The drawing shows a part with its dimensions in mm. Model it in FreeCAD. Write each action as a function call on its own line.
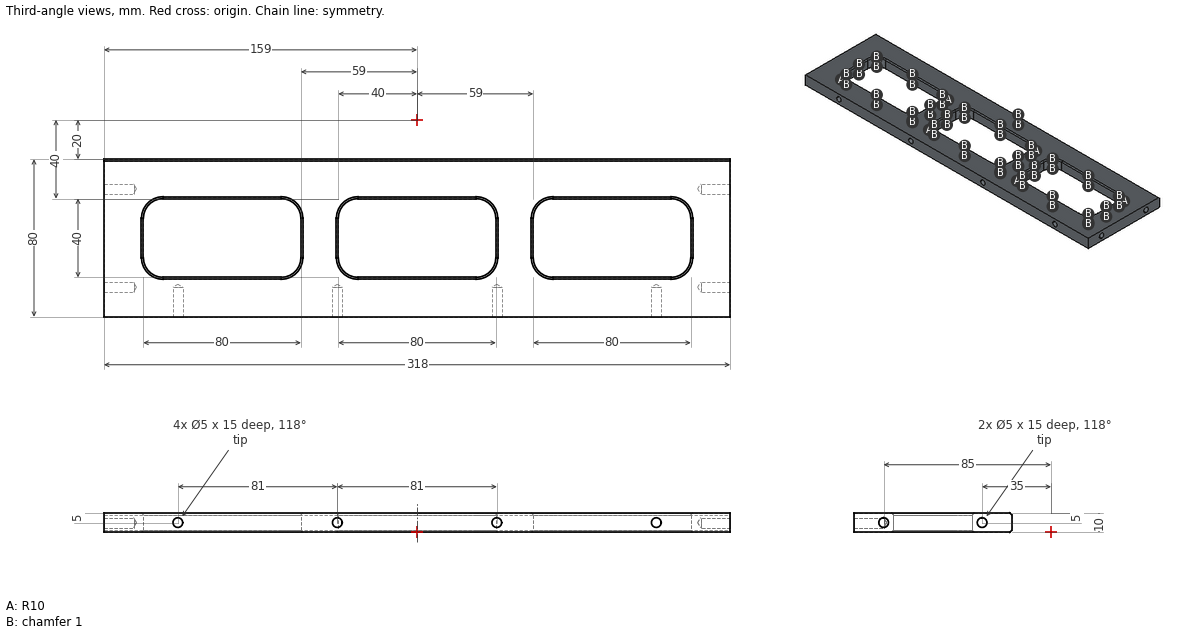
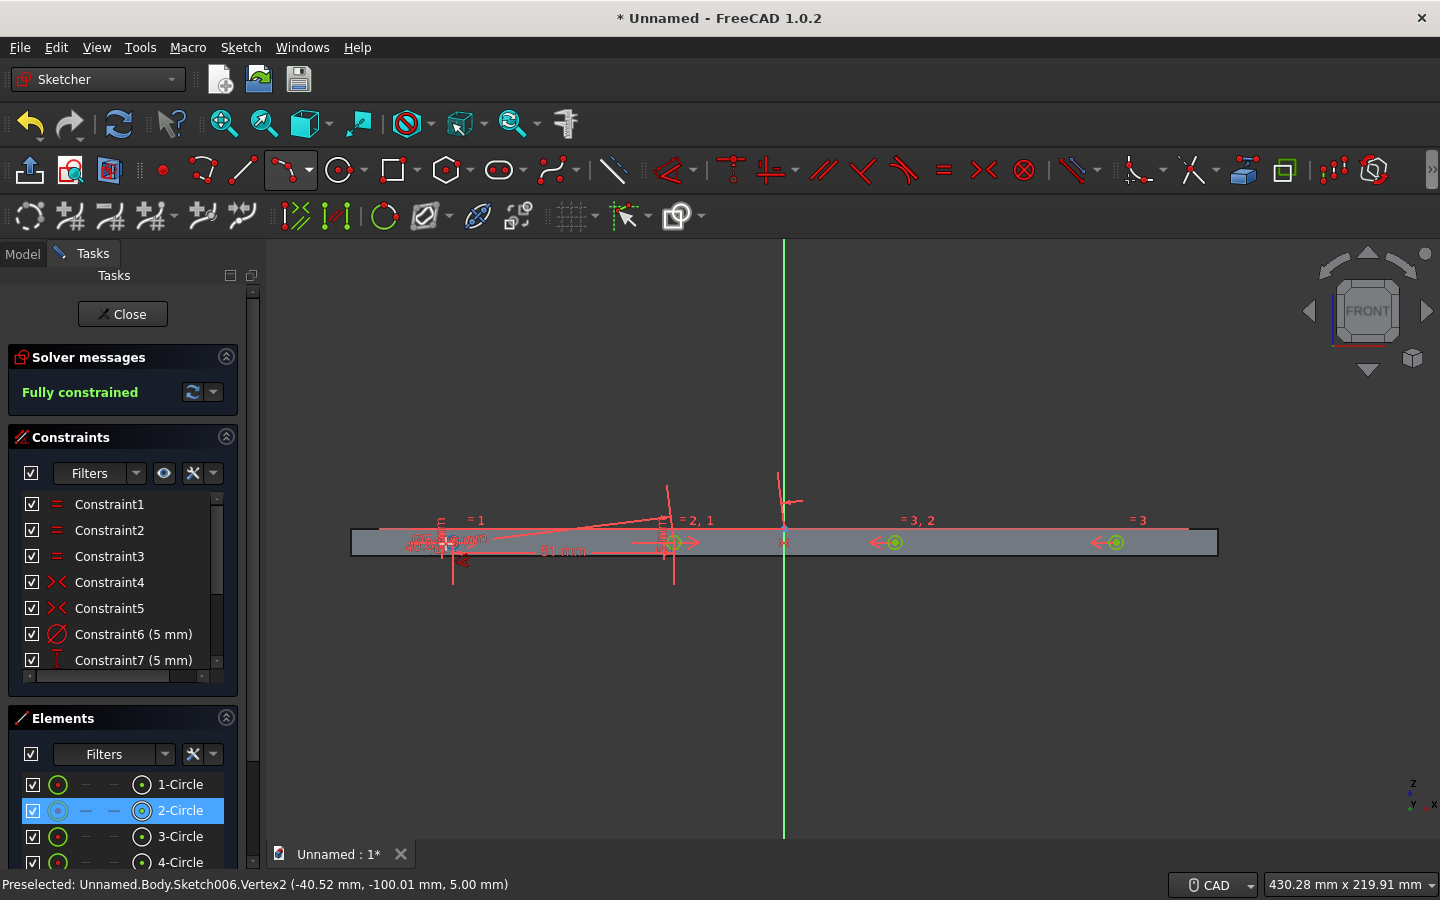
click(895, 543)
click(734, 577)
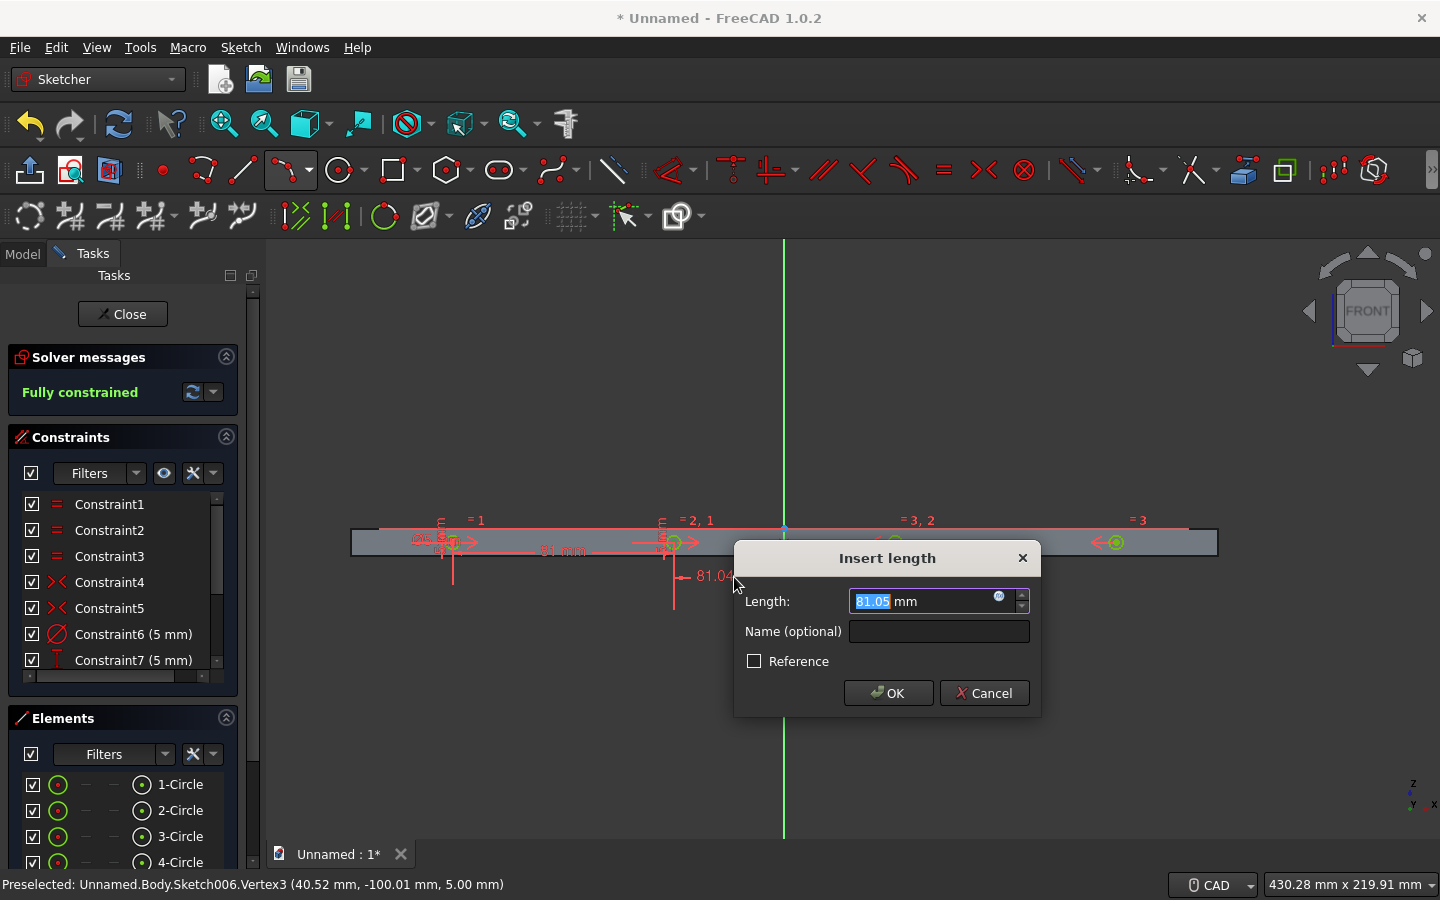
text(81)
key(Return)
key(Escape)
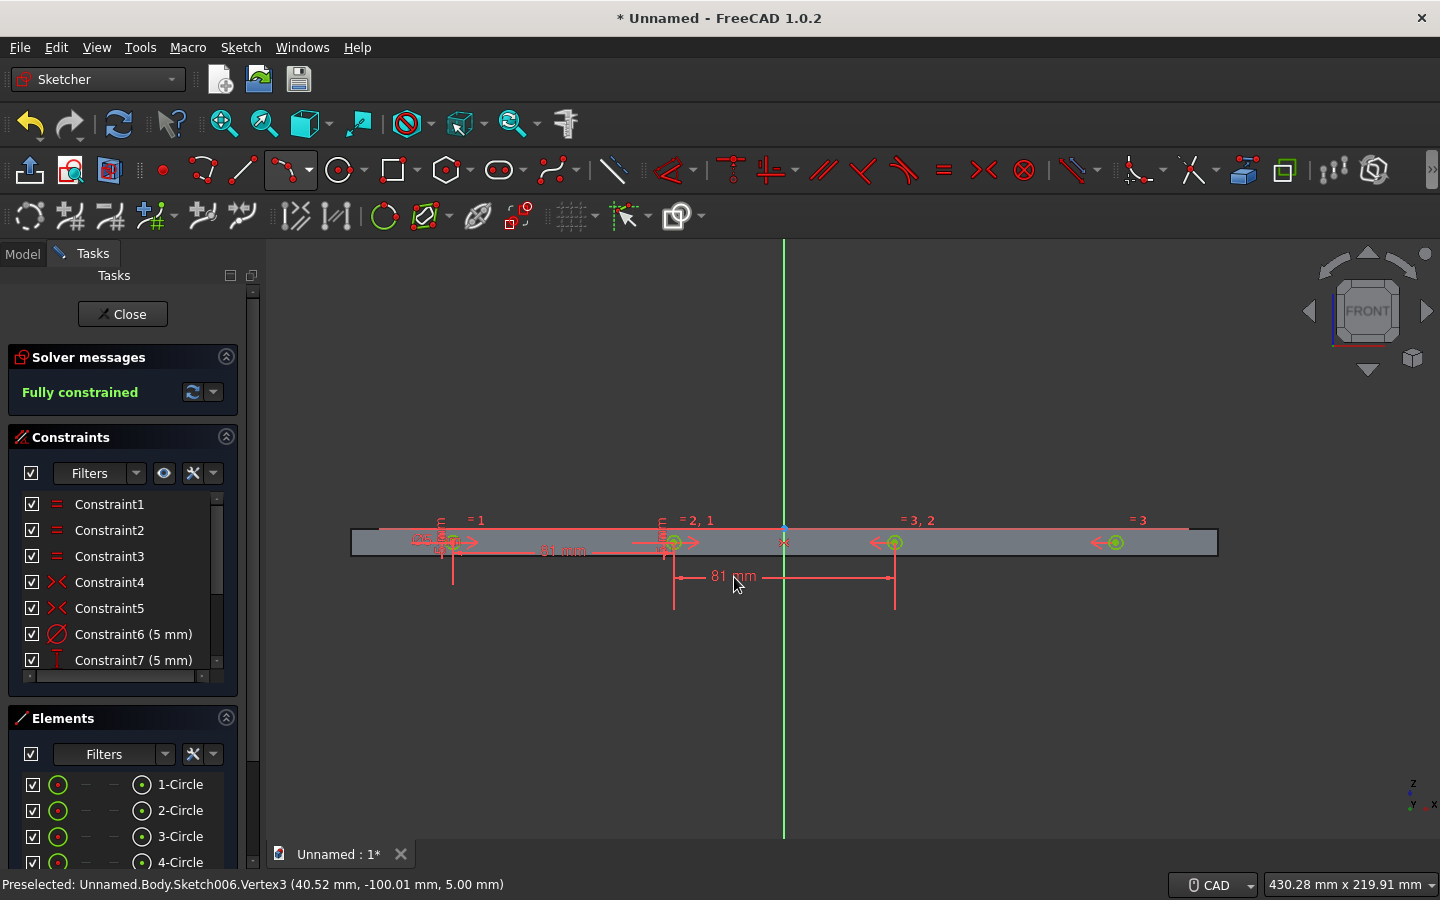
click(123, 314)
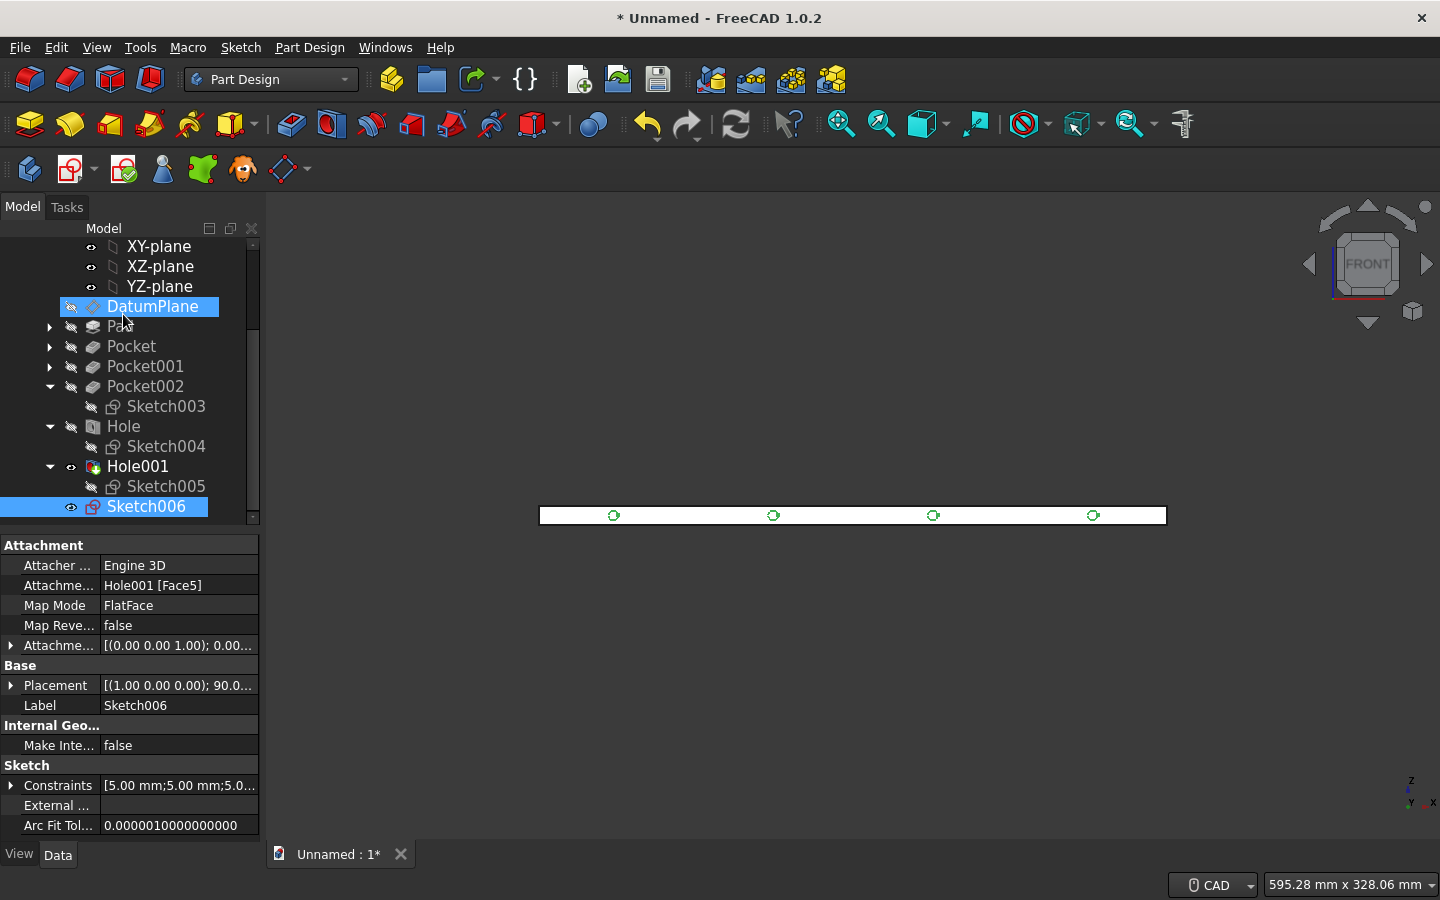
click(332, 124)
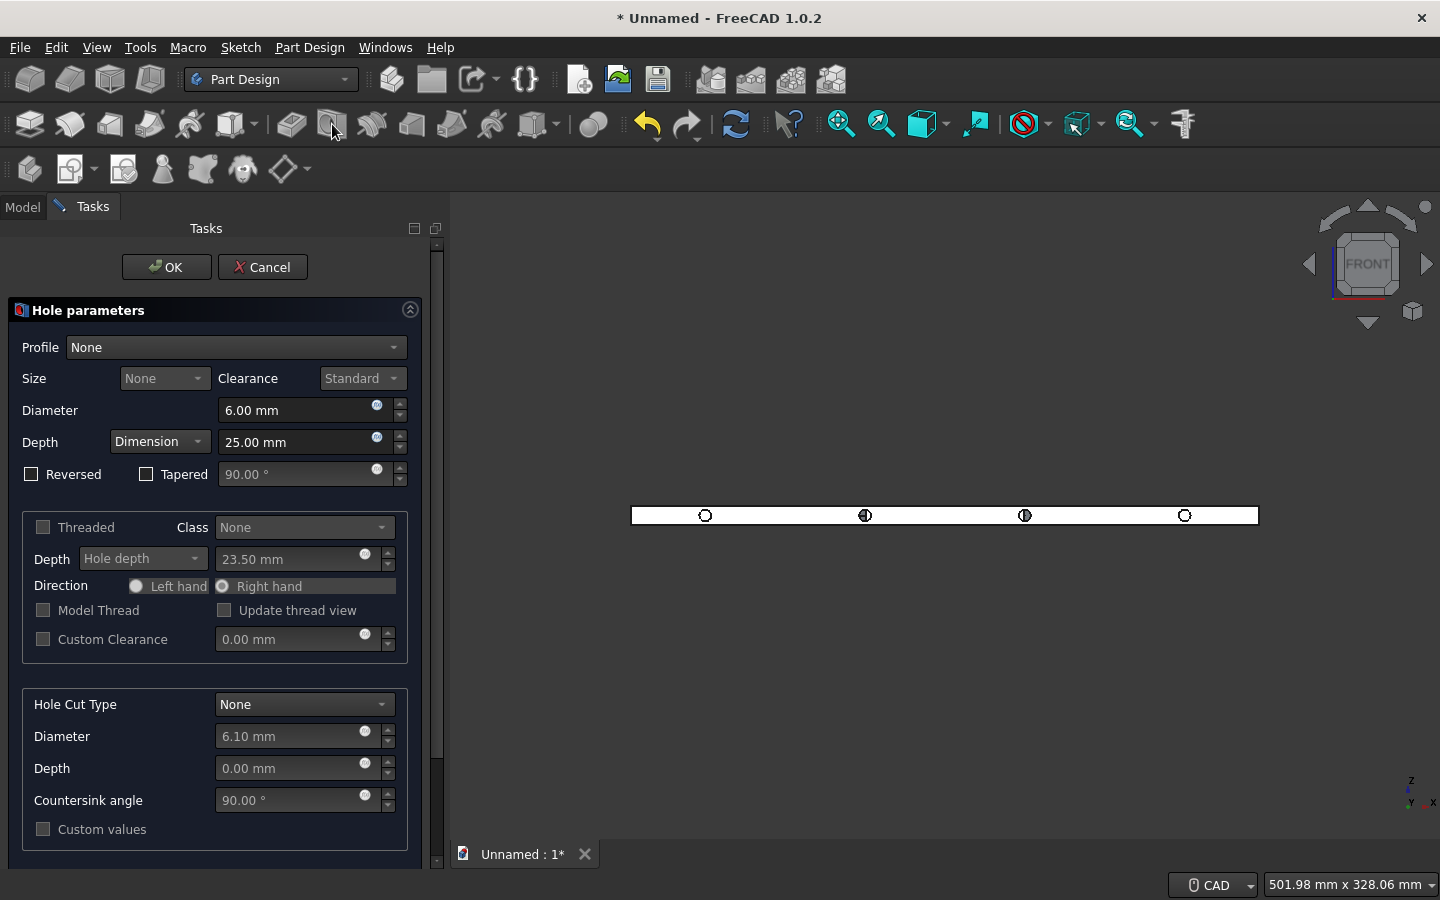
triple_click(305, 410)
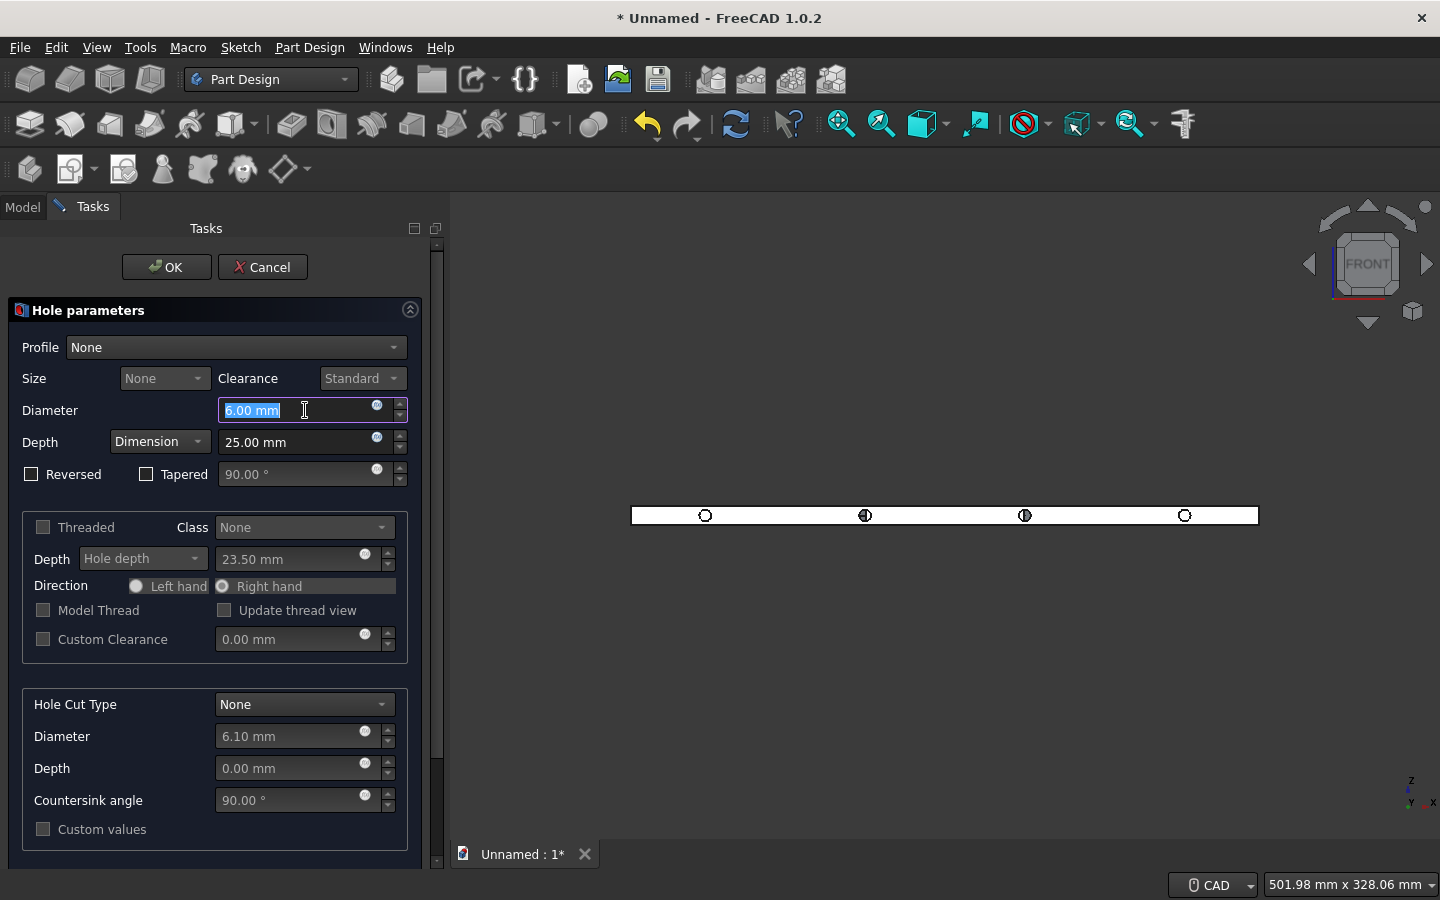
text(5)
key(Tab)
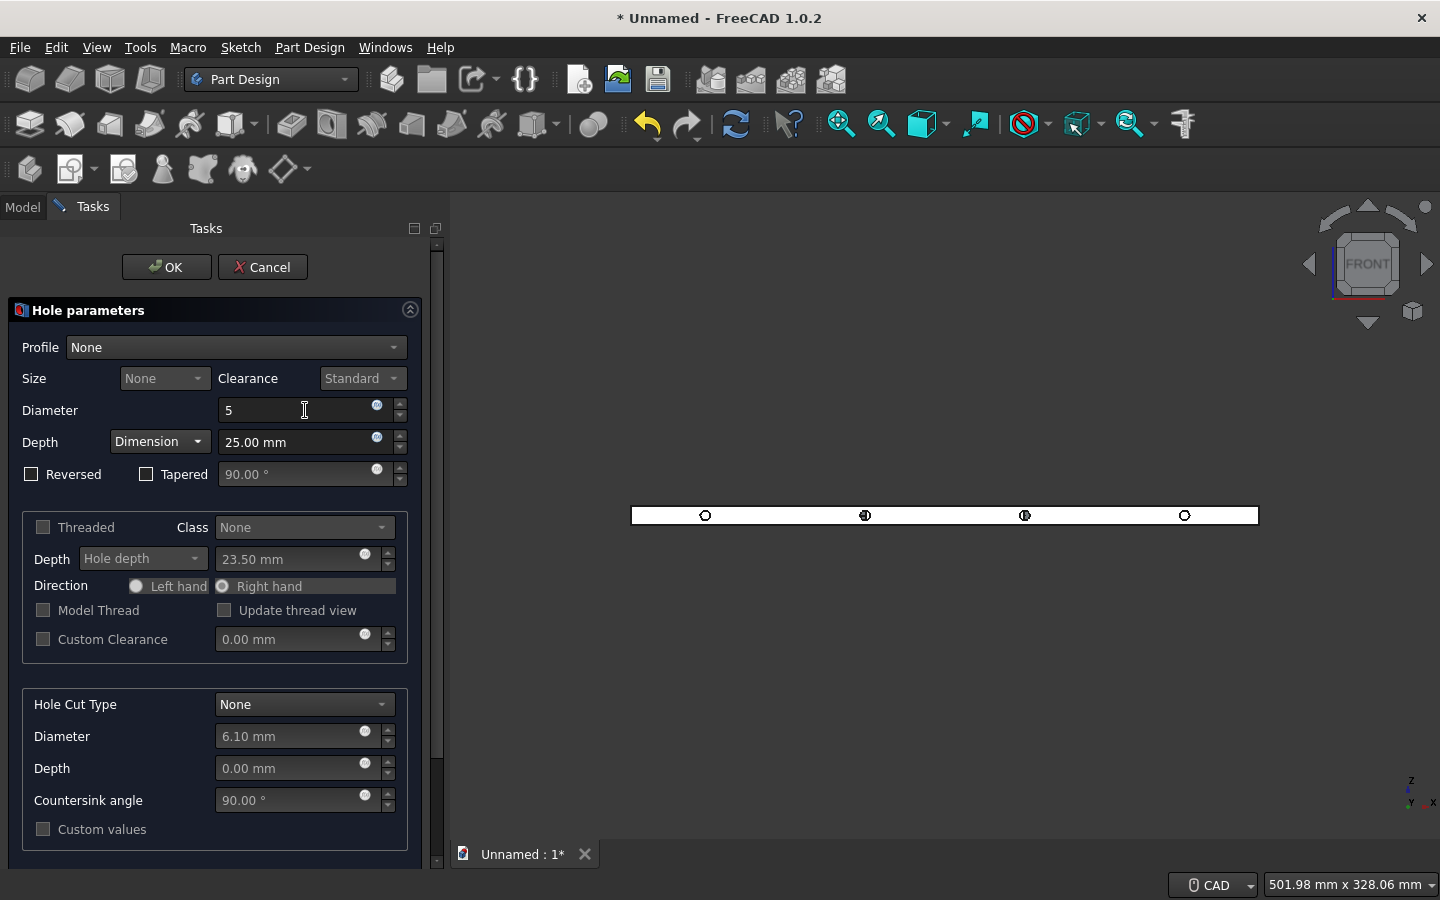
triple_click(305, 442)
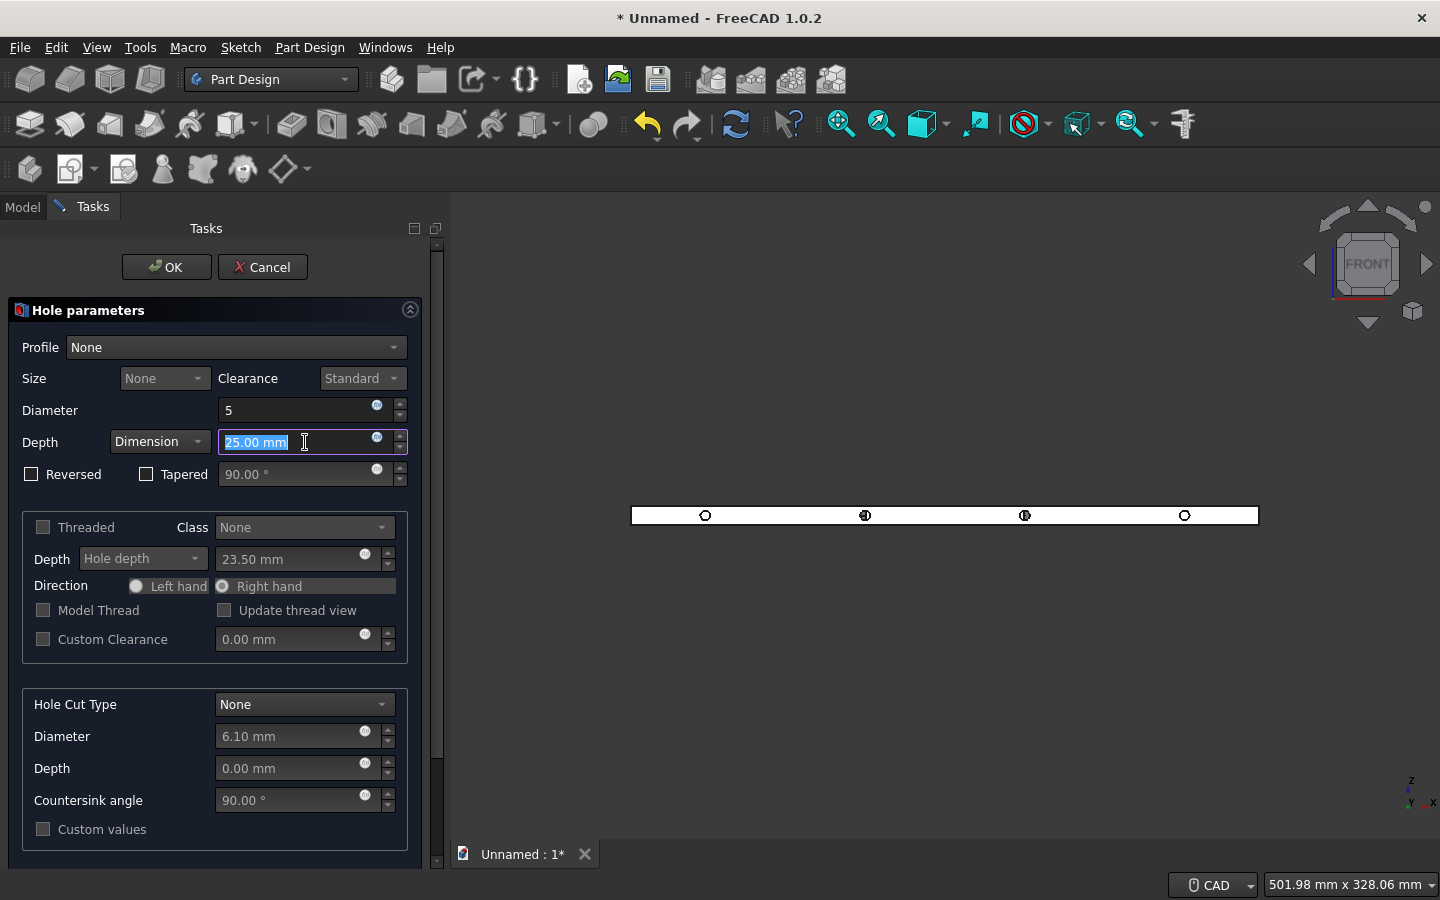
text(15)
key(Tab)